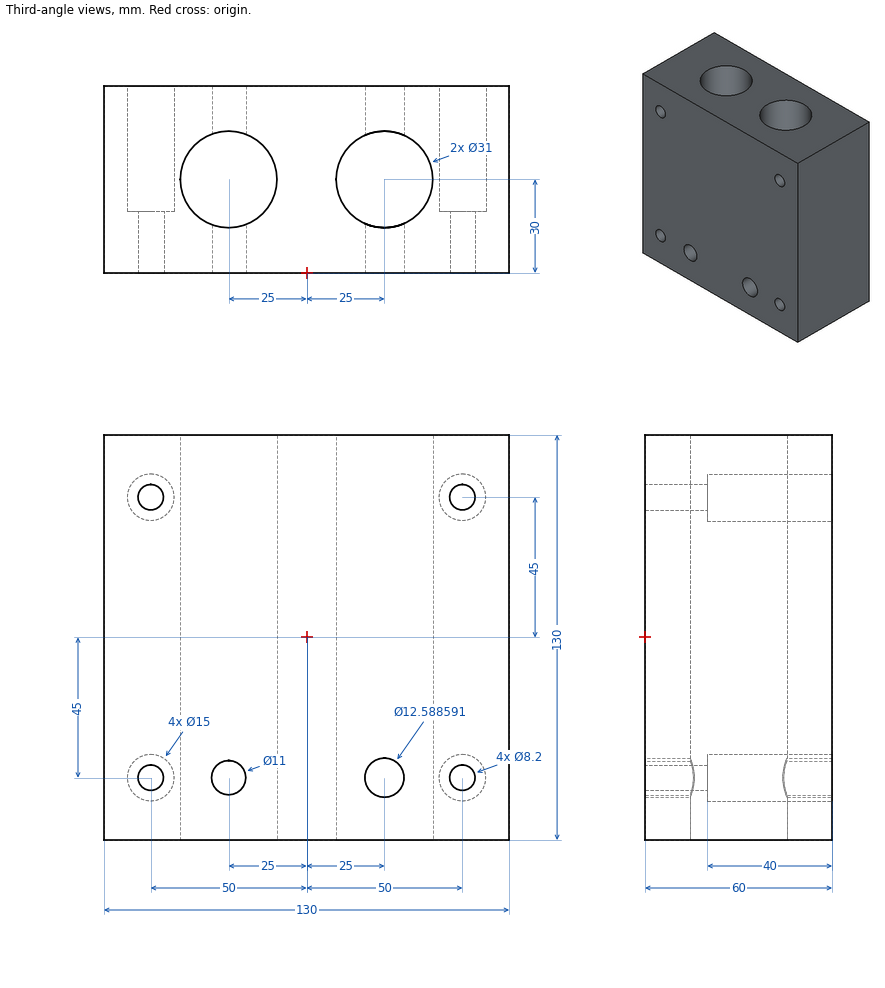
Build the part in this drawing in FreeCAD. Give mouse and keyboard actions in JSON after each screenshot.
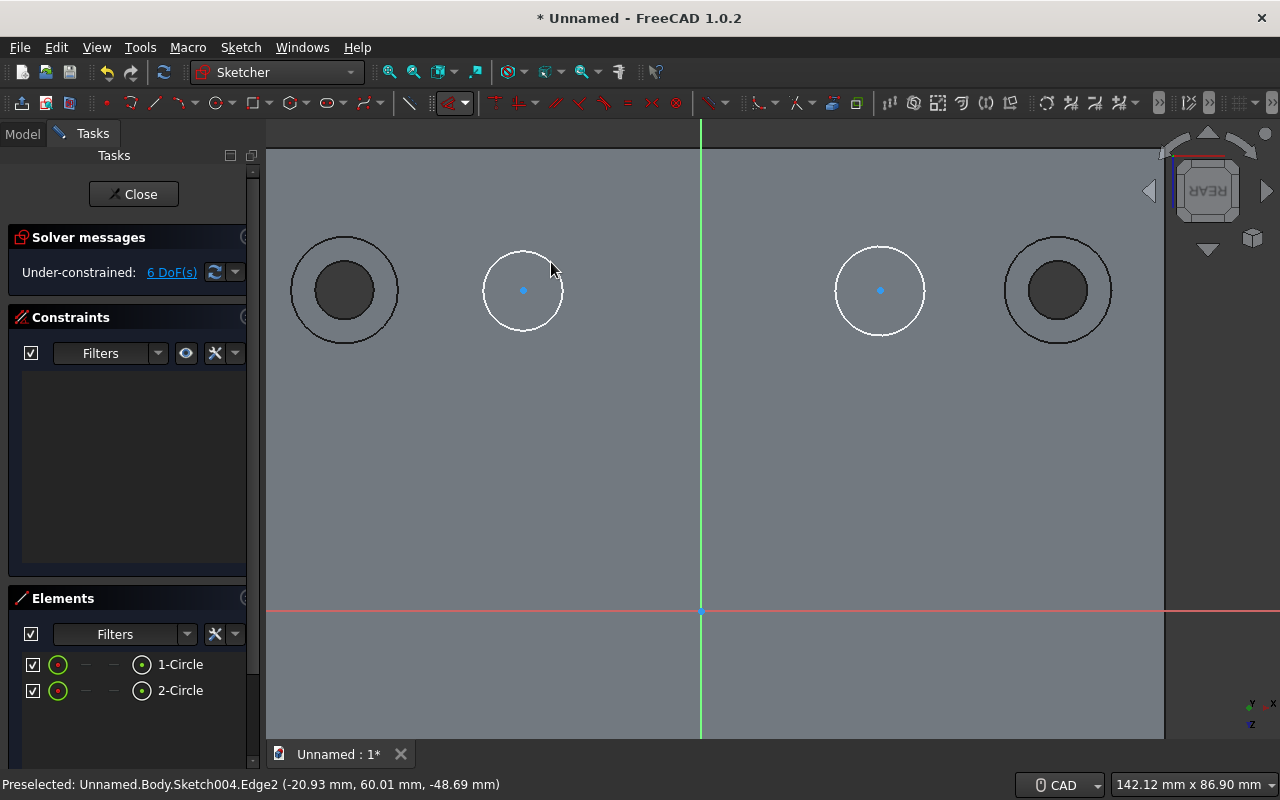
{"action": "left_click", "coordinate": [880, 291]}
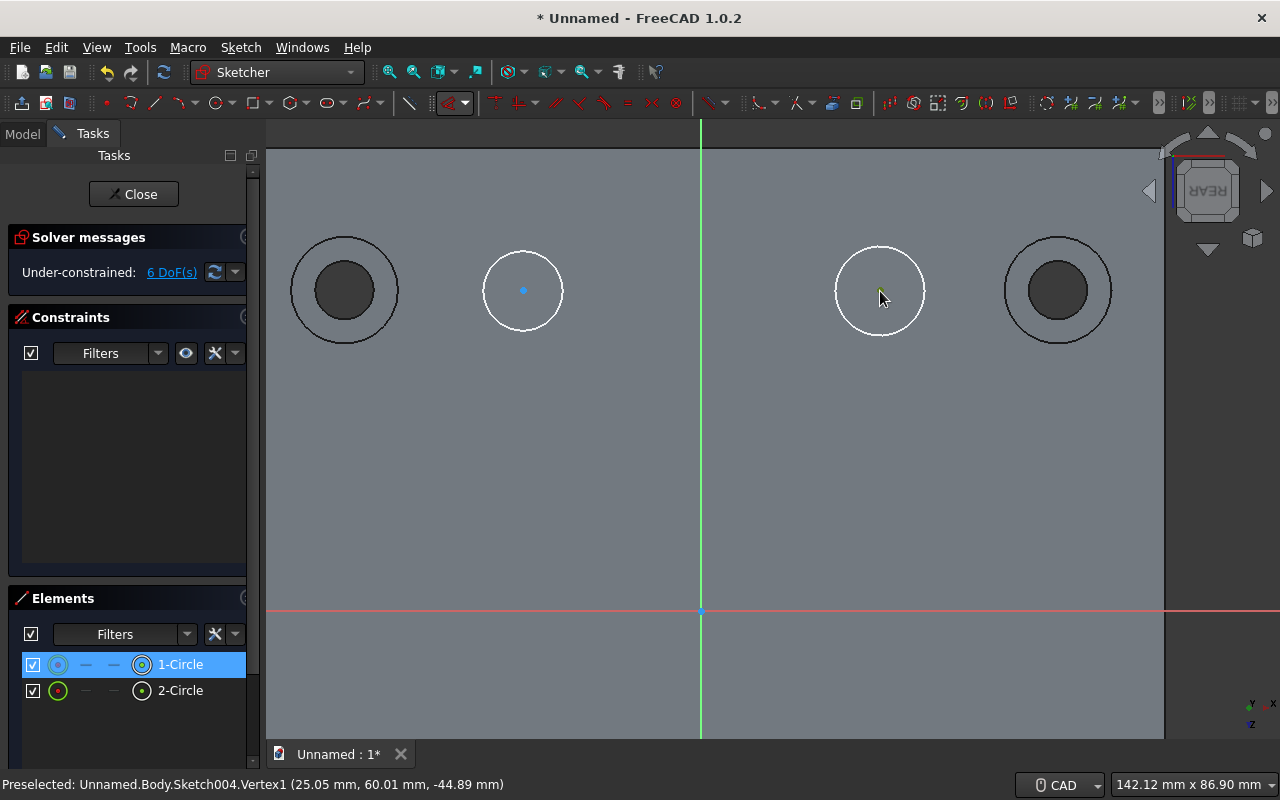
{"action": "left_click", "coordinate": [523, 291]}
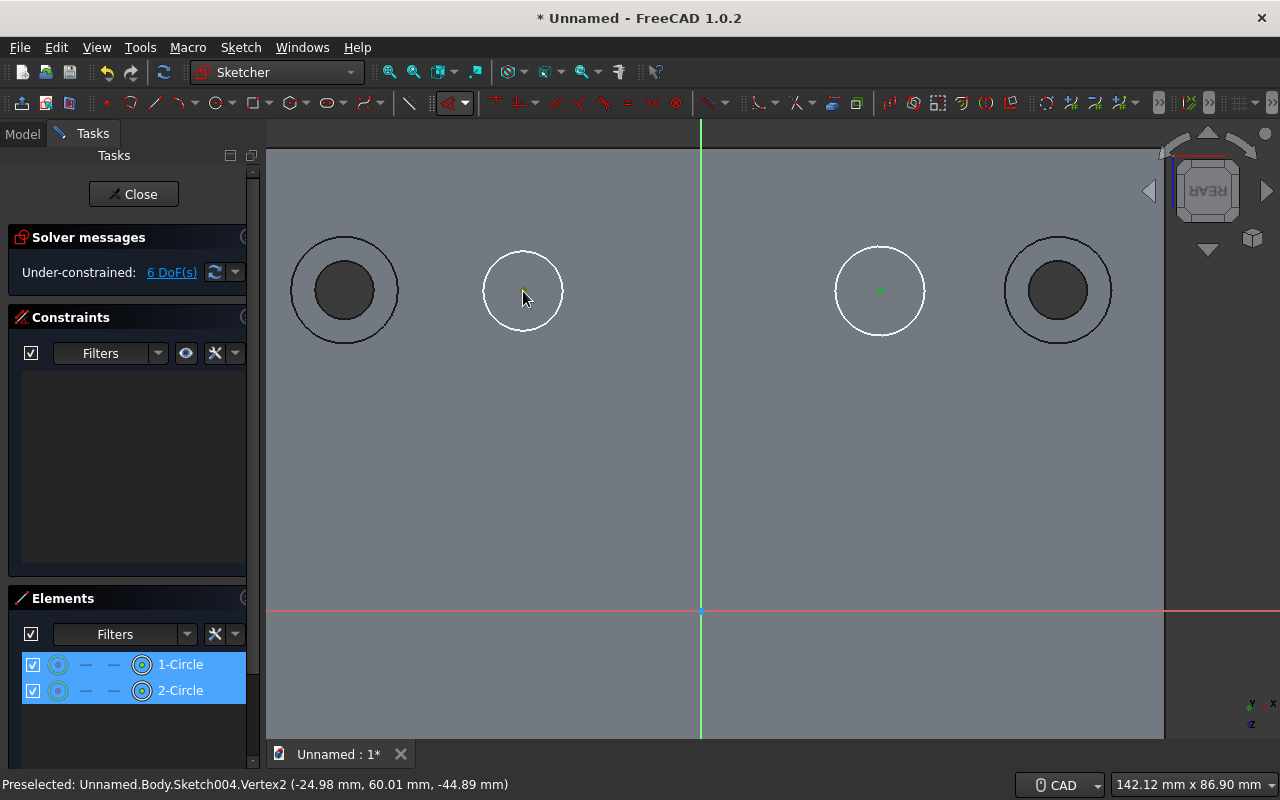
{"action": "key", "text": "h"}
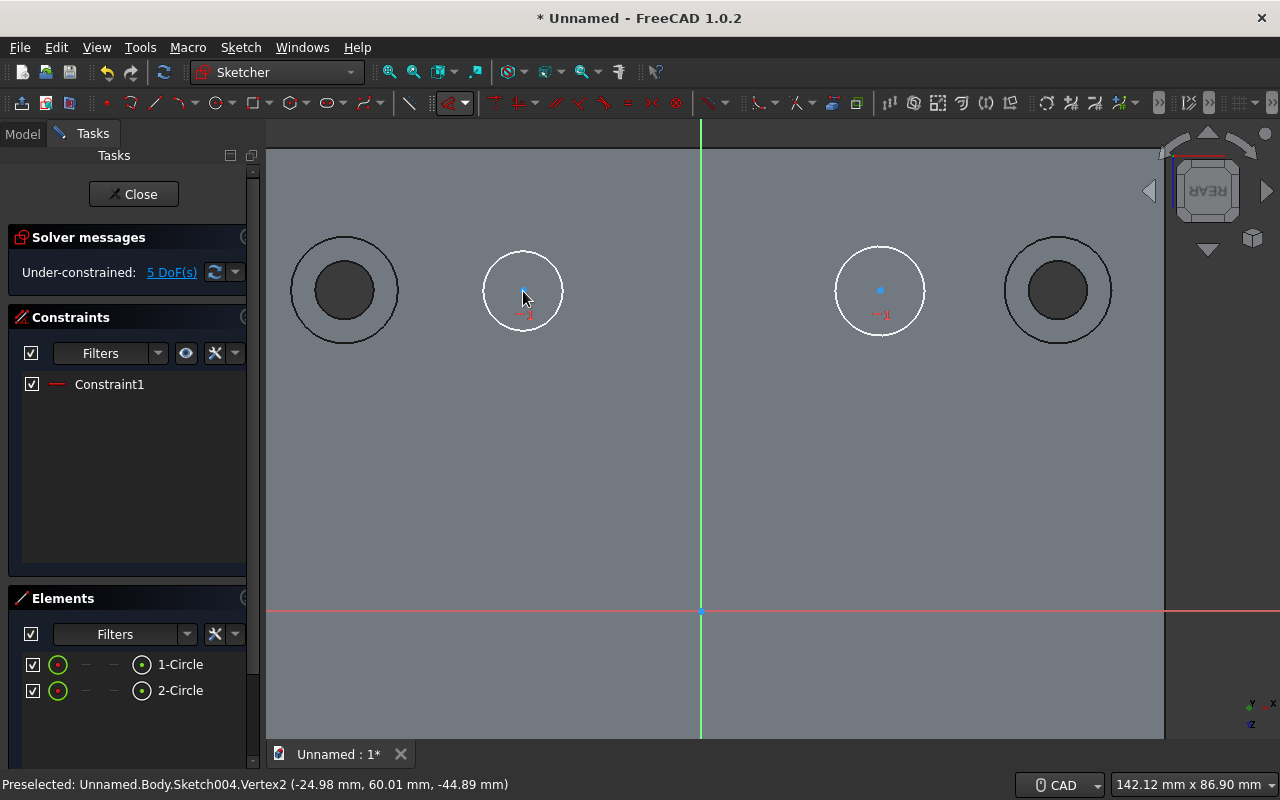
{"action": "left_click", "coordinate": [911, 259]}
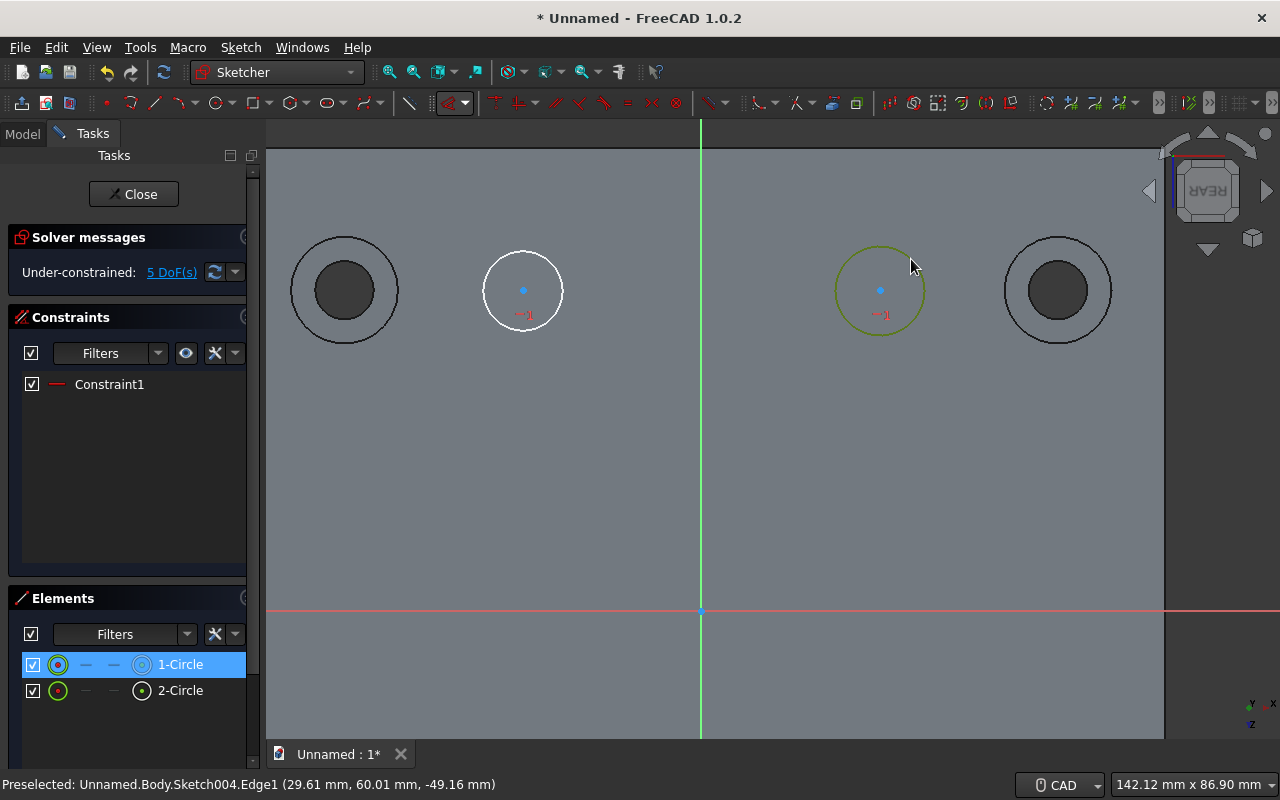
{"action": "key", "text": "k o"}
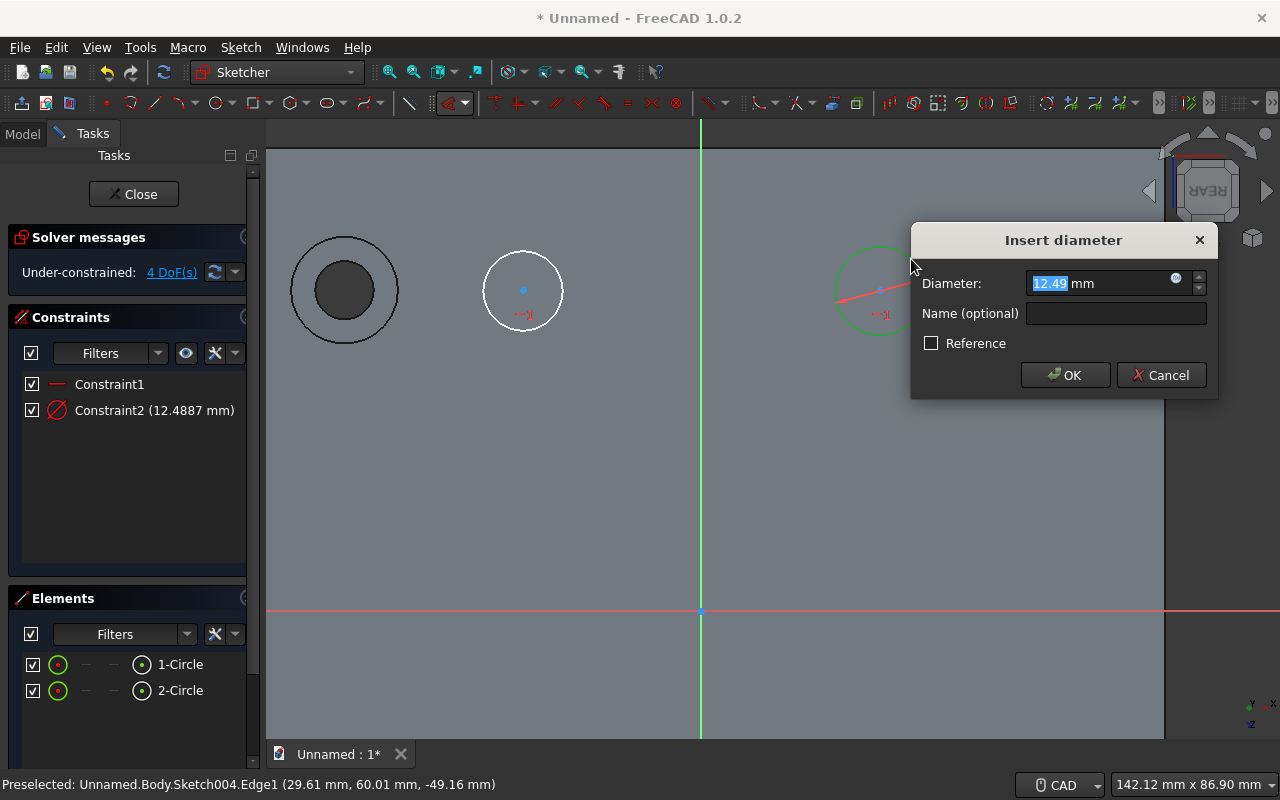
{"action": "type", "text": "12.588591"}
{"action": "key", "text": "Return"}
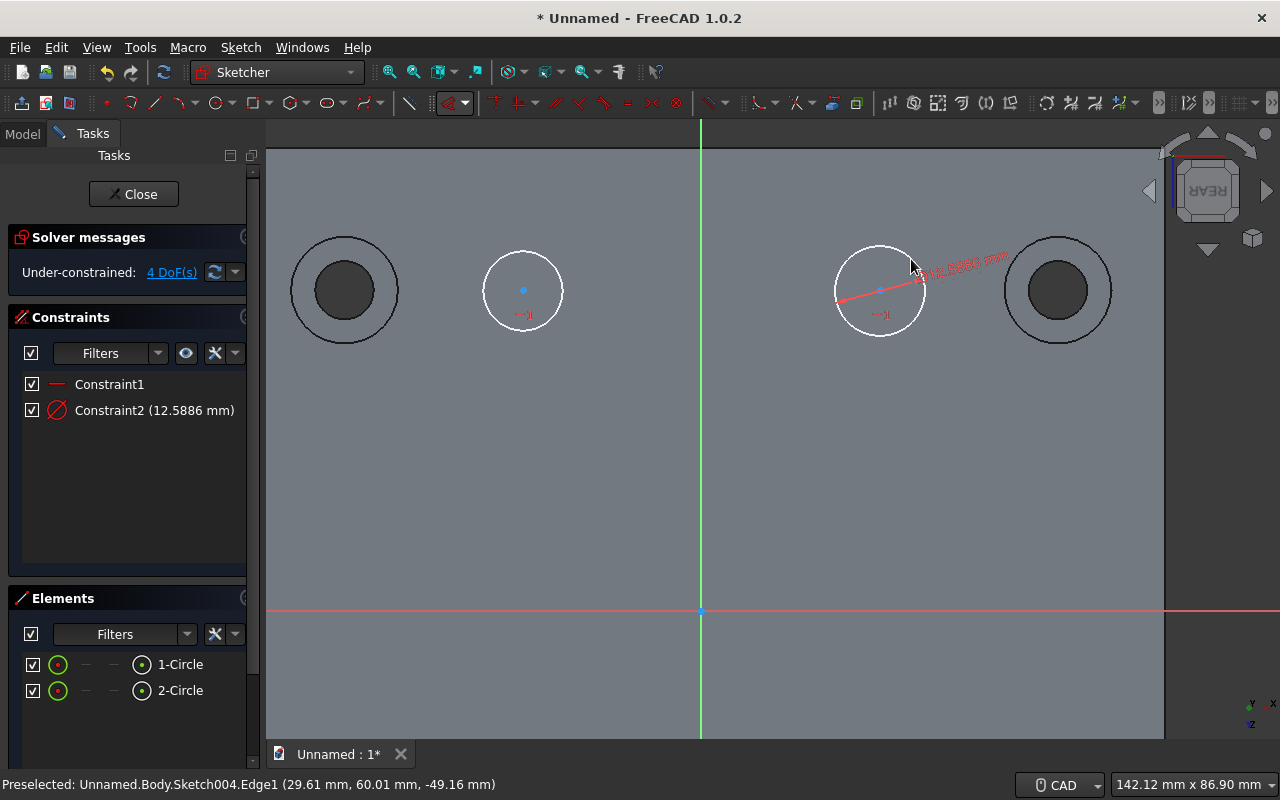
{"action": "left_click", "coordinate": [551, 263]}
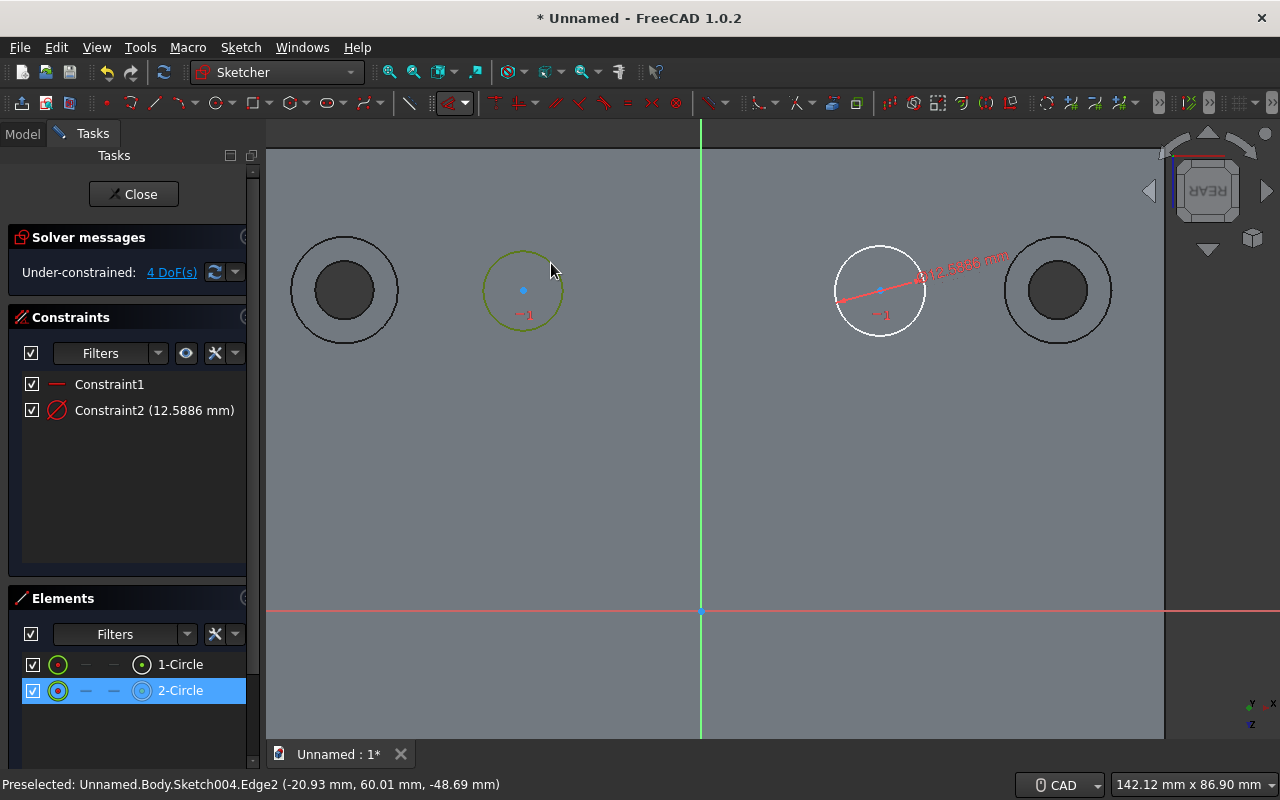
{"action": "left_click", "coordinate": [468, 104]}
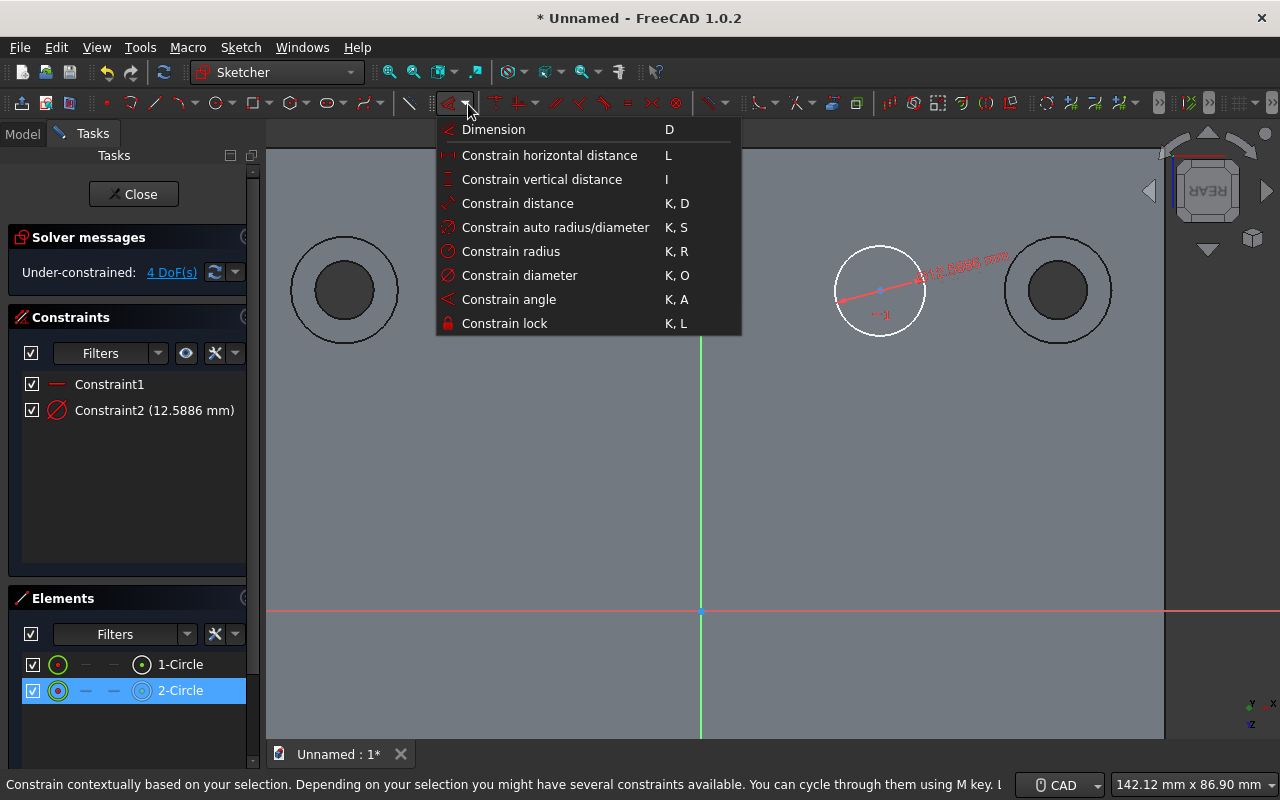
{"action": "left_click", "coordinate": [589, 275]}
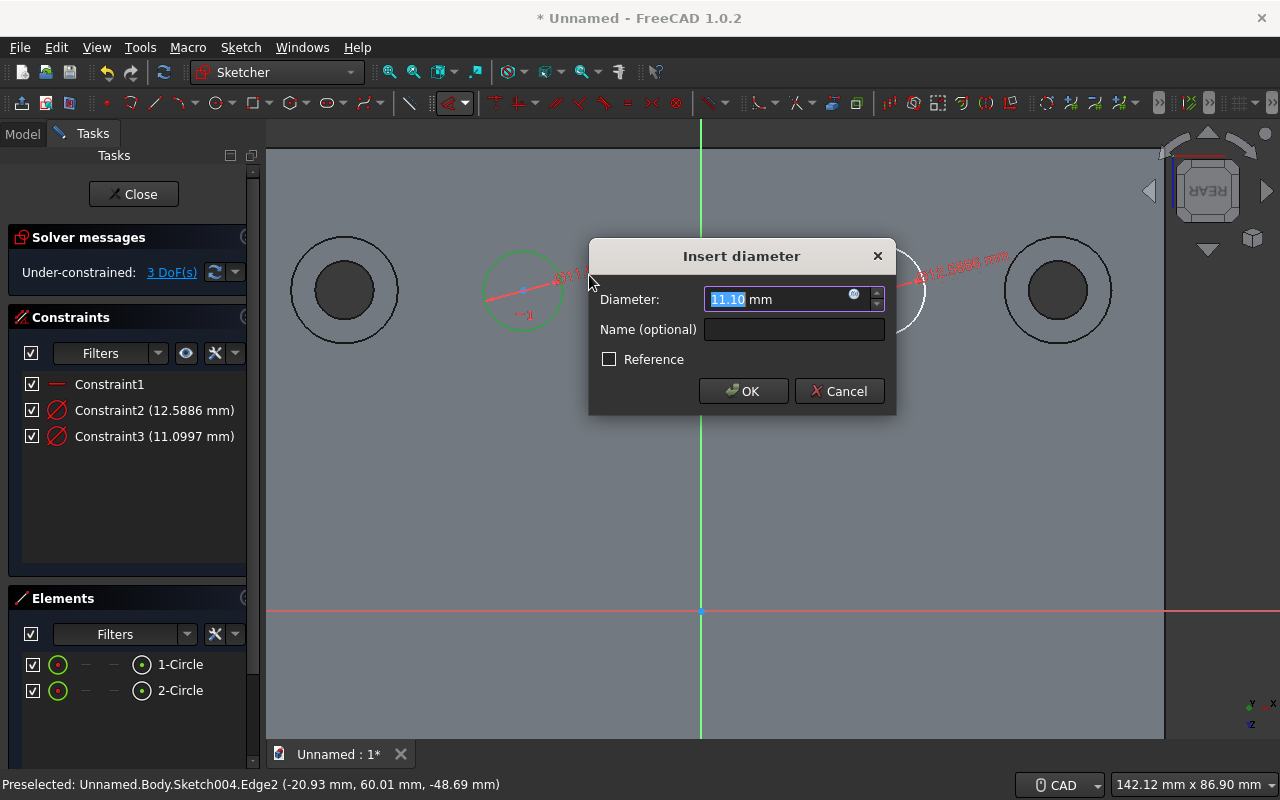
{"action": "type", "text": "11"}
{"action": "key", "text": "Return"}